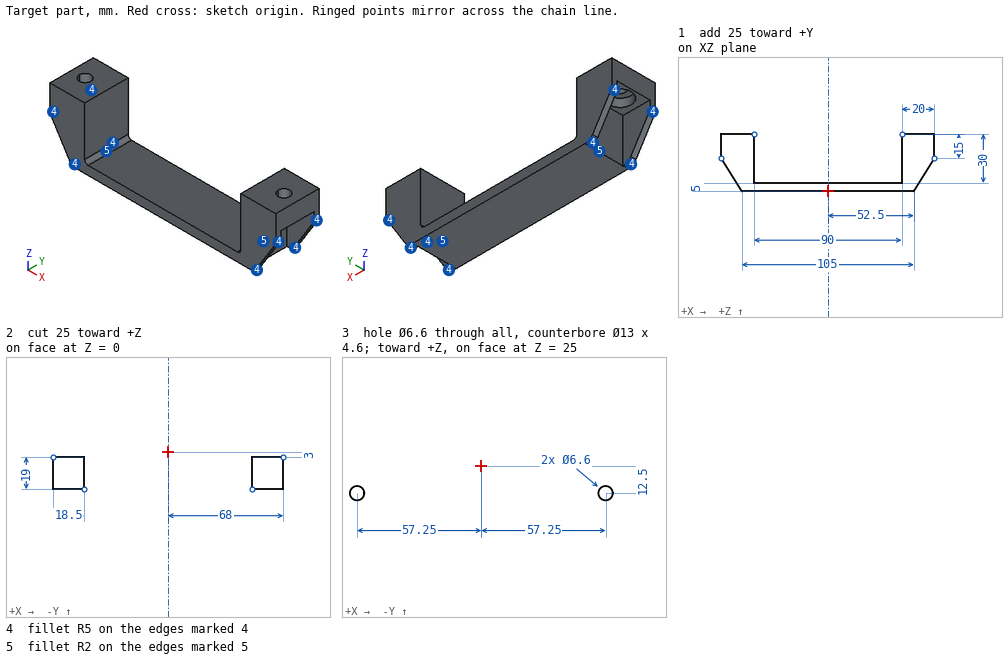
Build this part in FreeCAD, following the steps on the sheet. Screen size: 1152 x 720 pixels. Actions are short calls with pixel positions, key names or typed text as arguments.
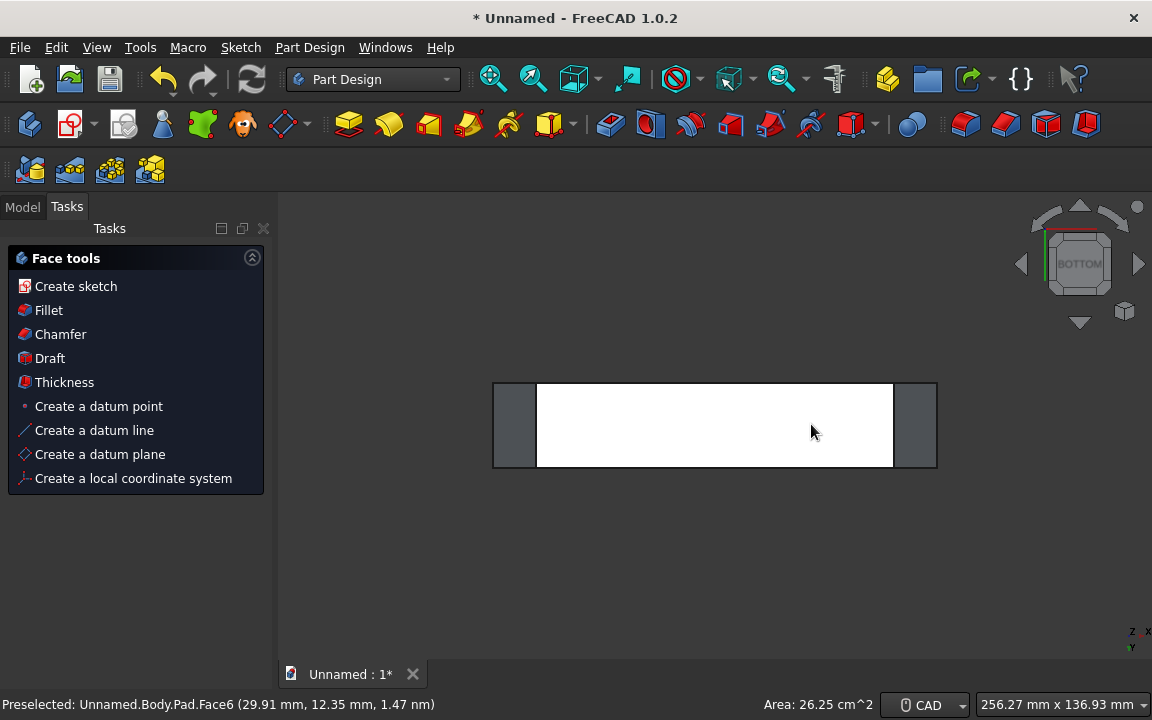
click(70, 124)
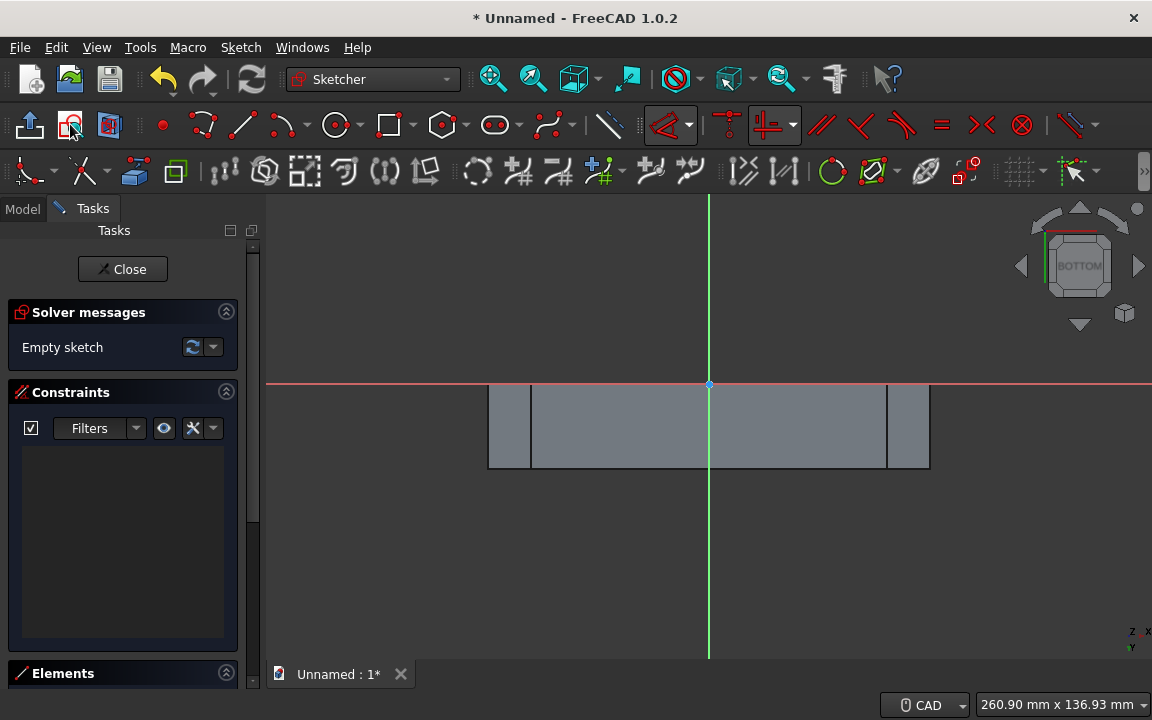
click(390, 126)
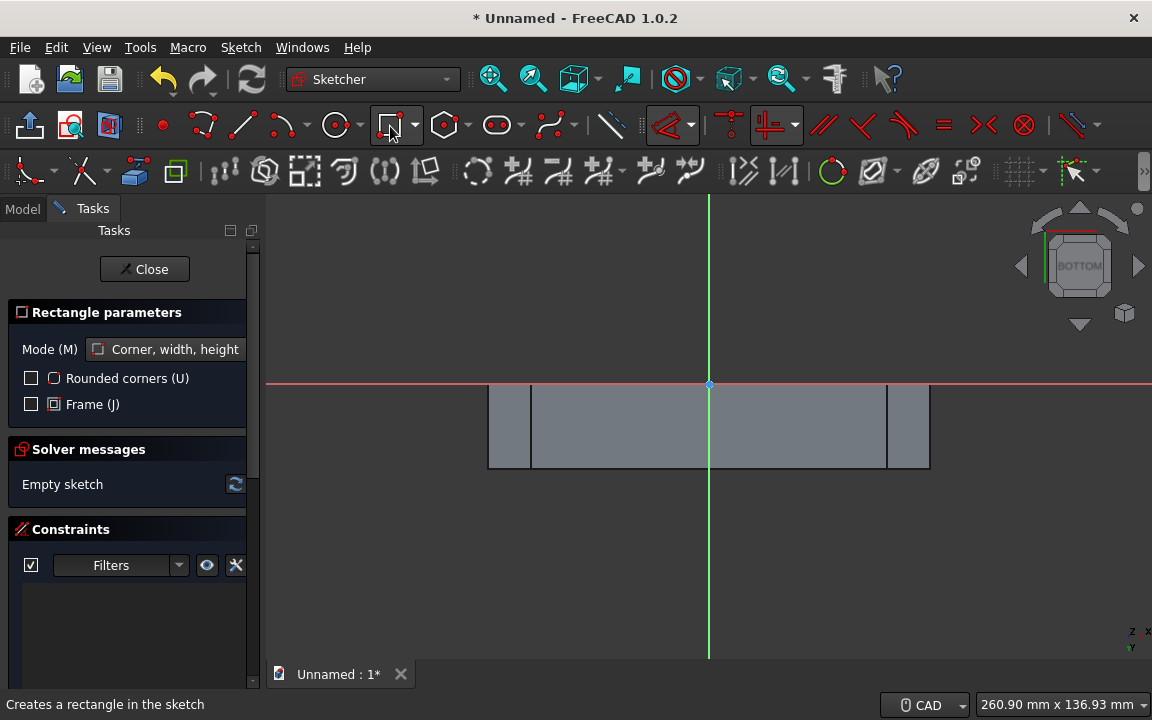
scroll(877, 394, up, 3)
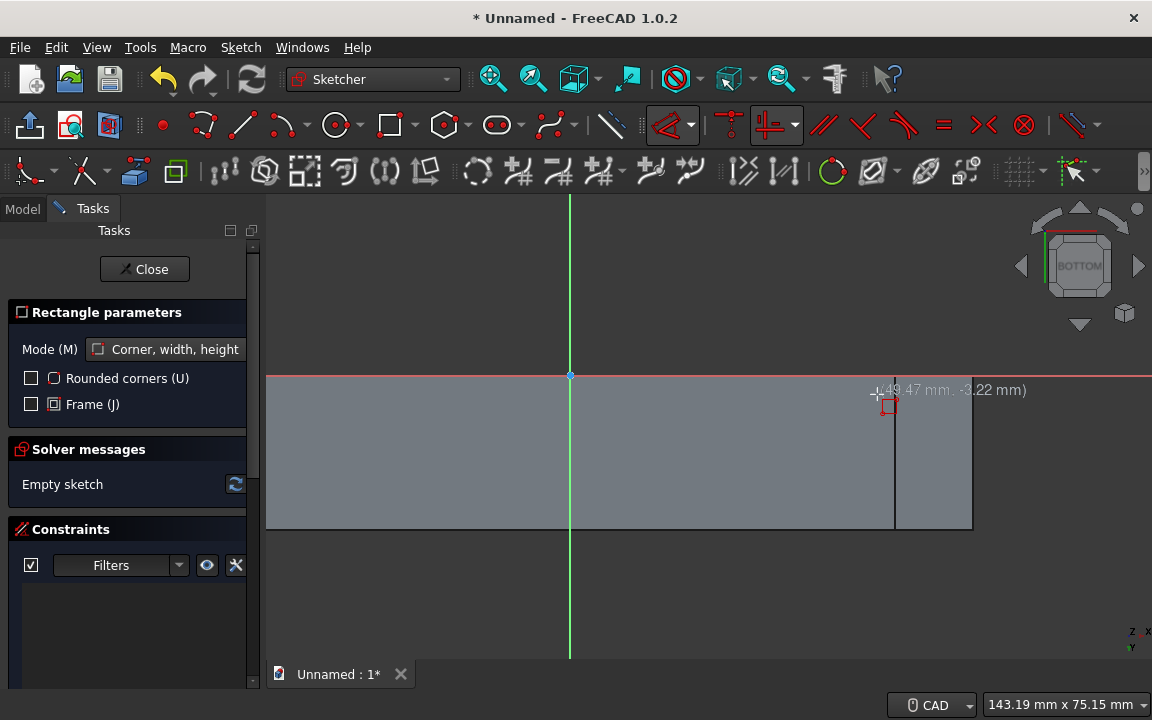
click(877, 394)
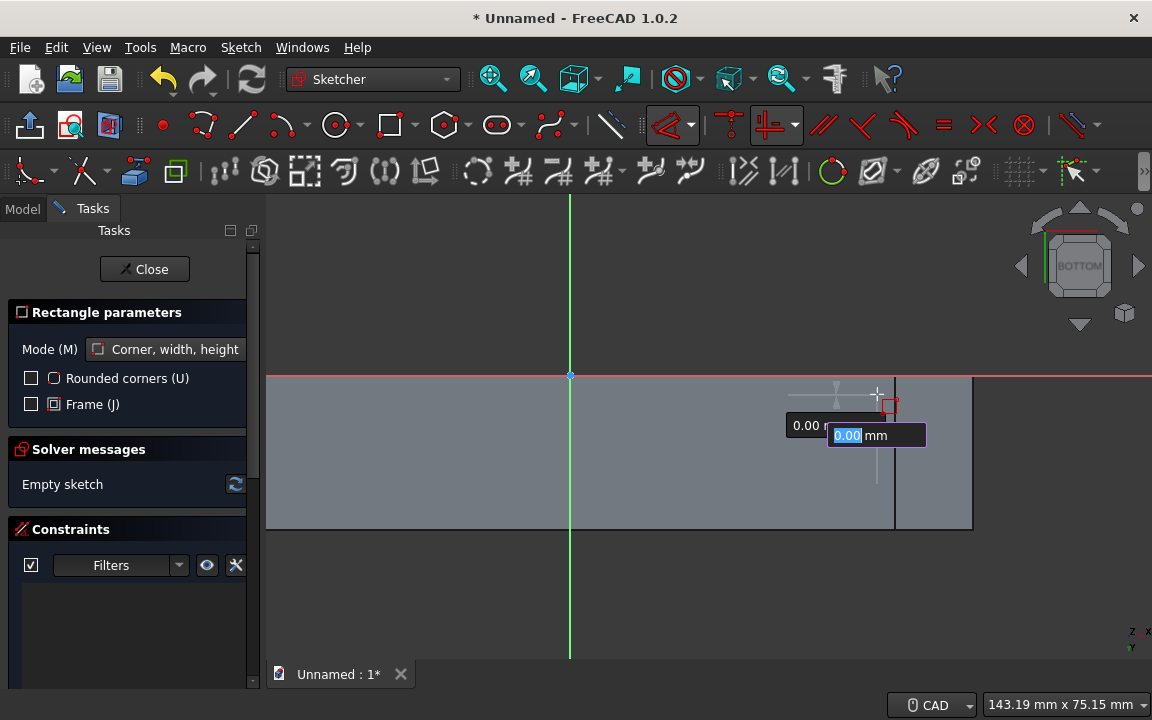
scroll(726, 406, down, 3)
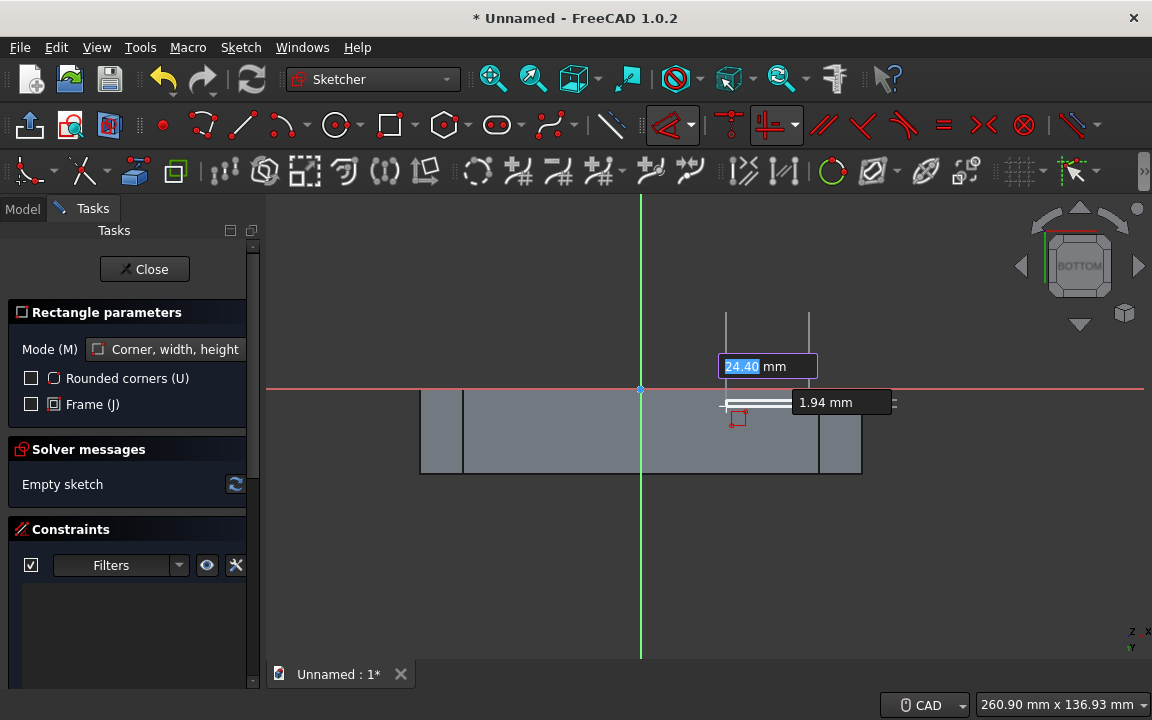
click(872, 464)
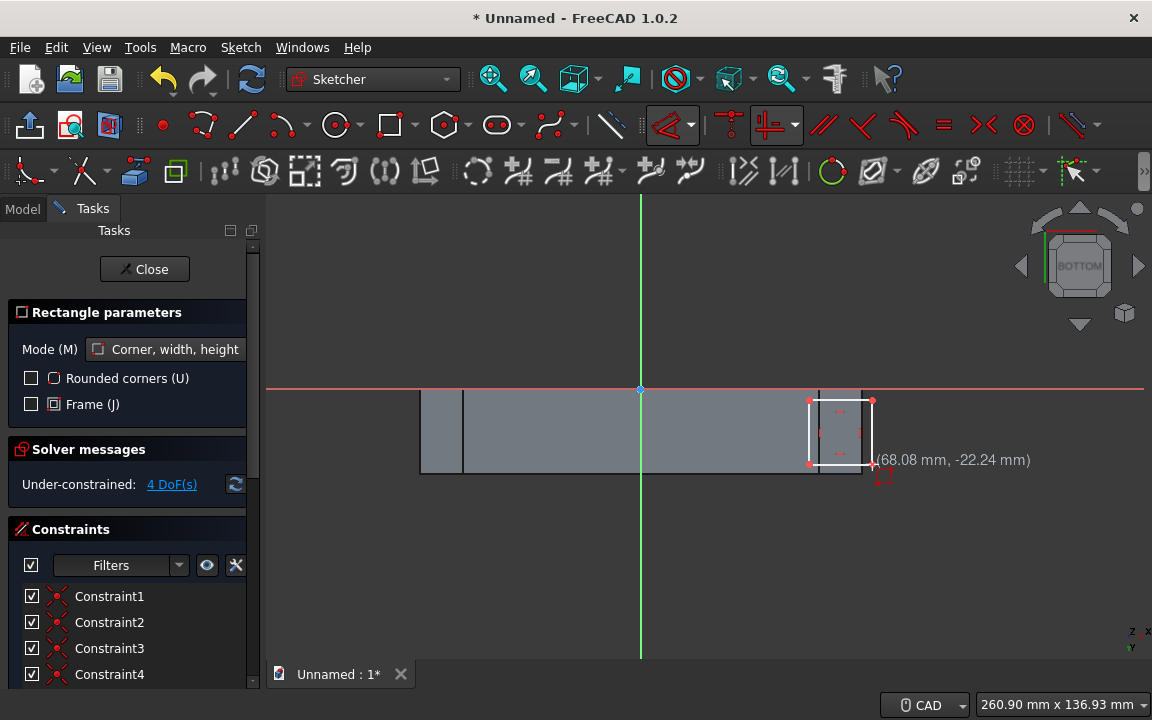
scroll(410, 400, up, 3)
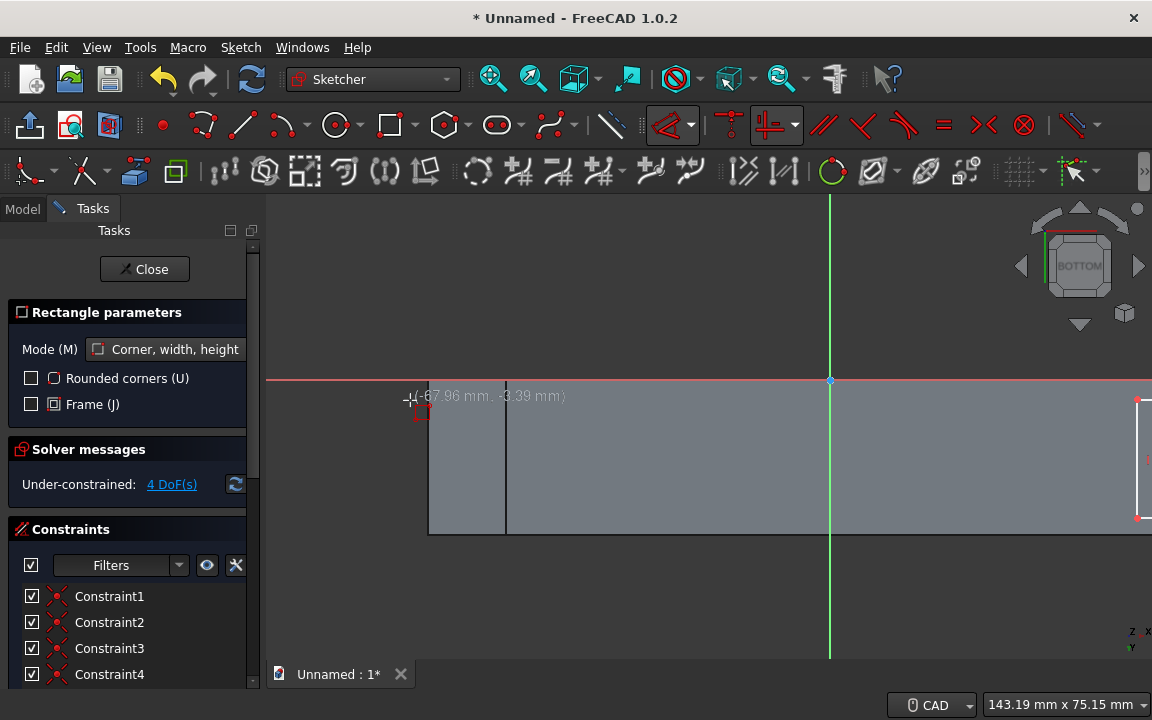
click(410, 399)
move(524, 517)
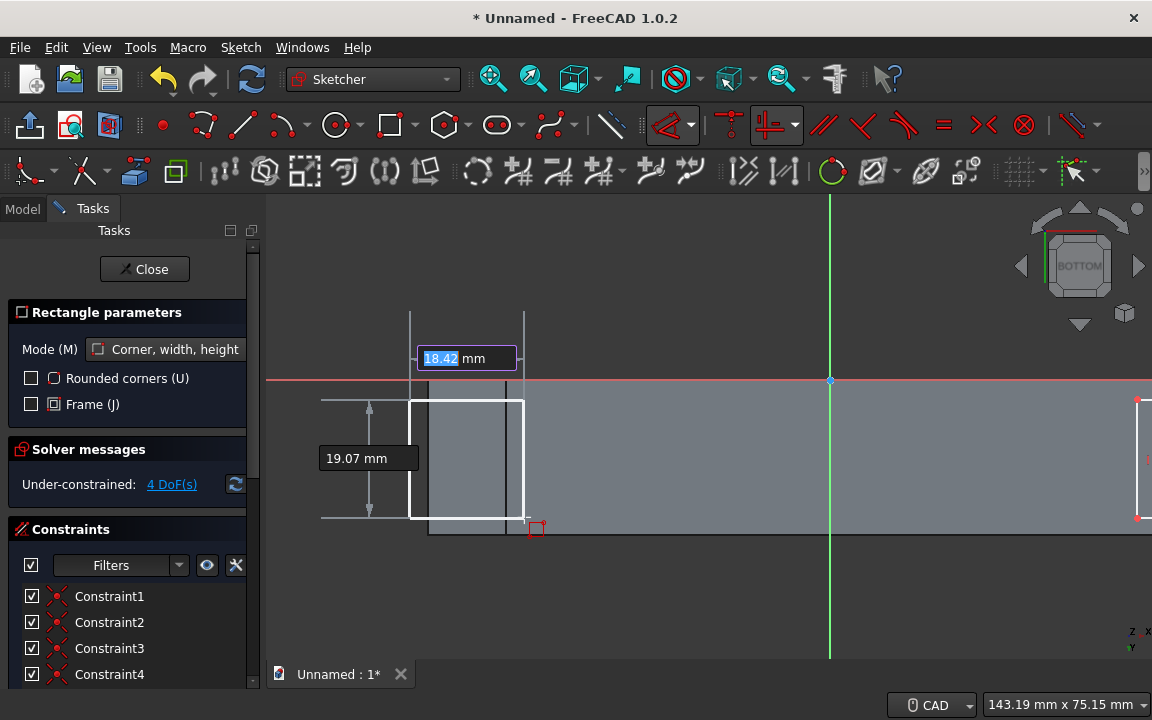
text(18.5)
key(Tab)
text(19)
key(Return)
key(Escape)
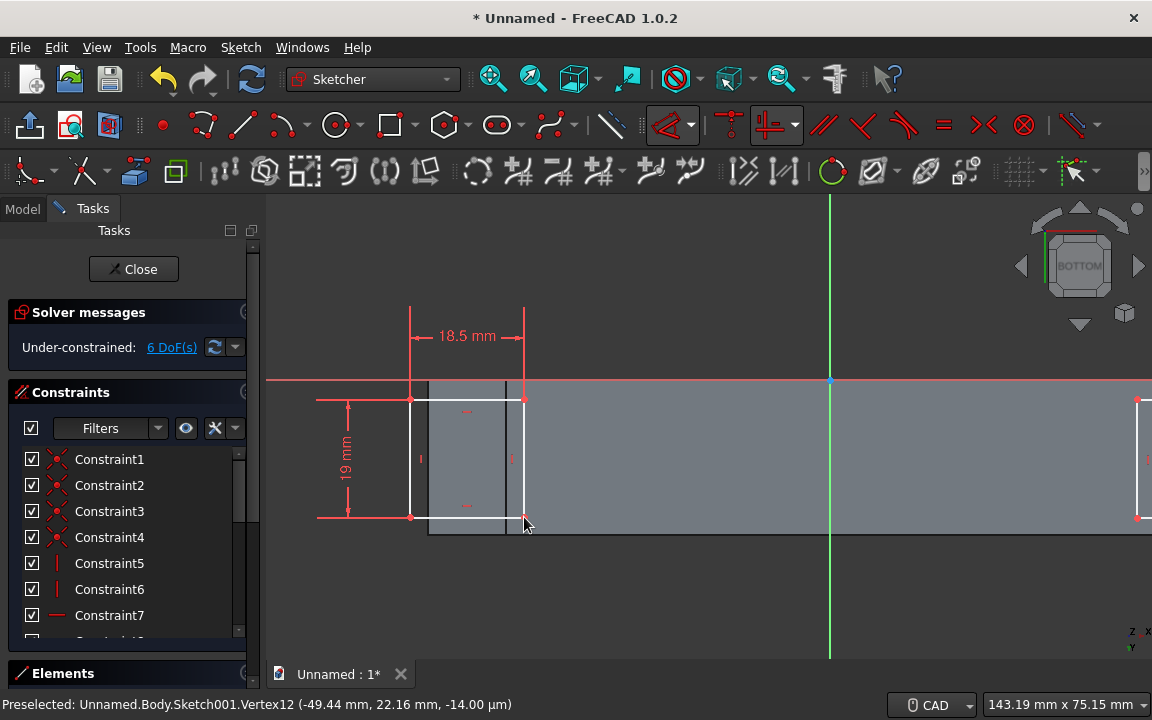
scroll(410, 400, down, 3)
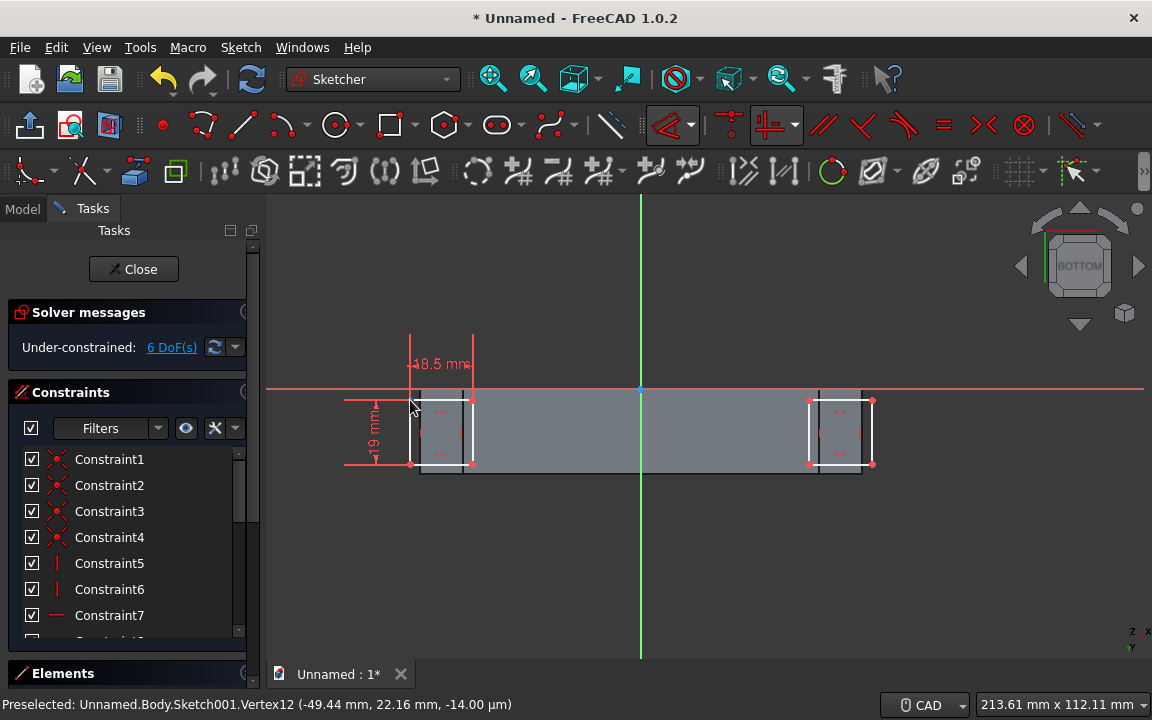
click(872, 400)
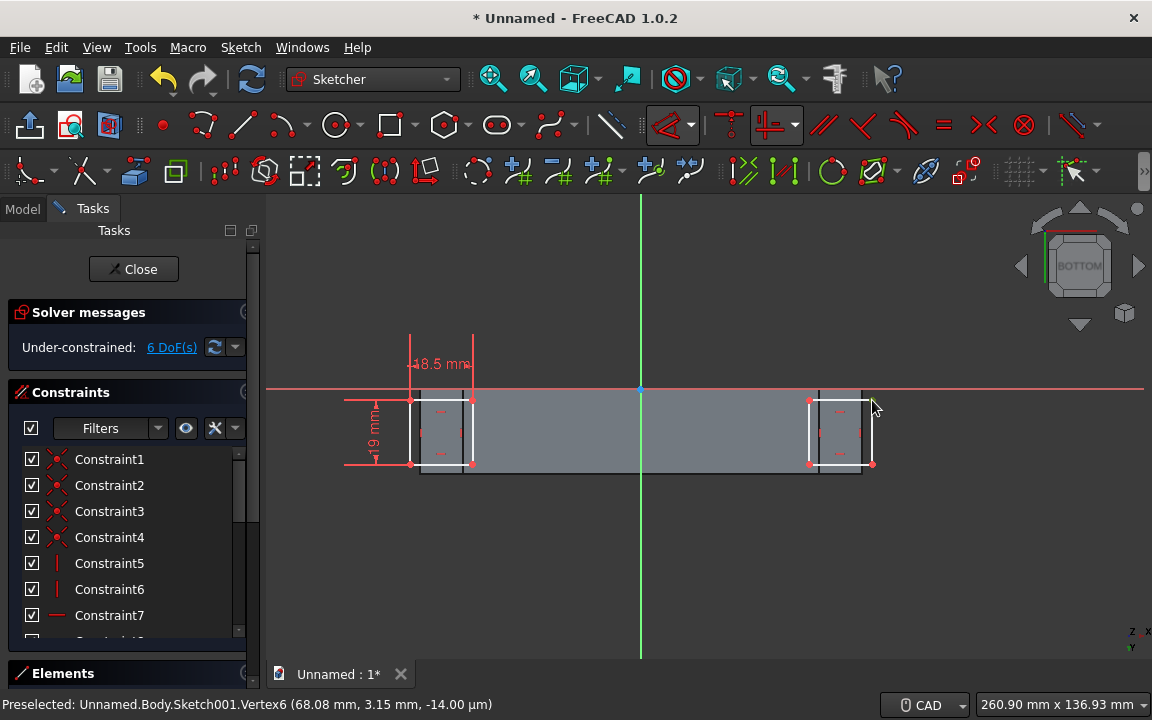
click(410, 400)